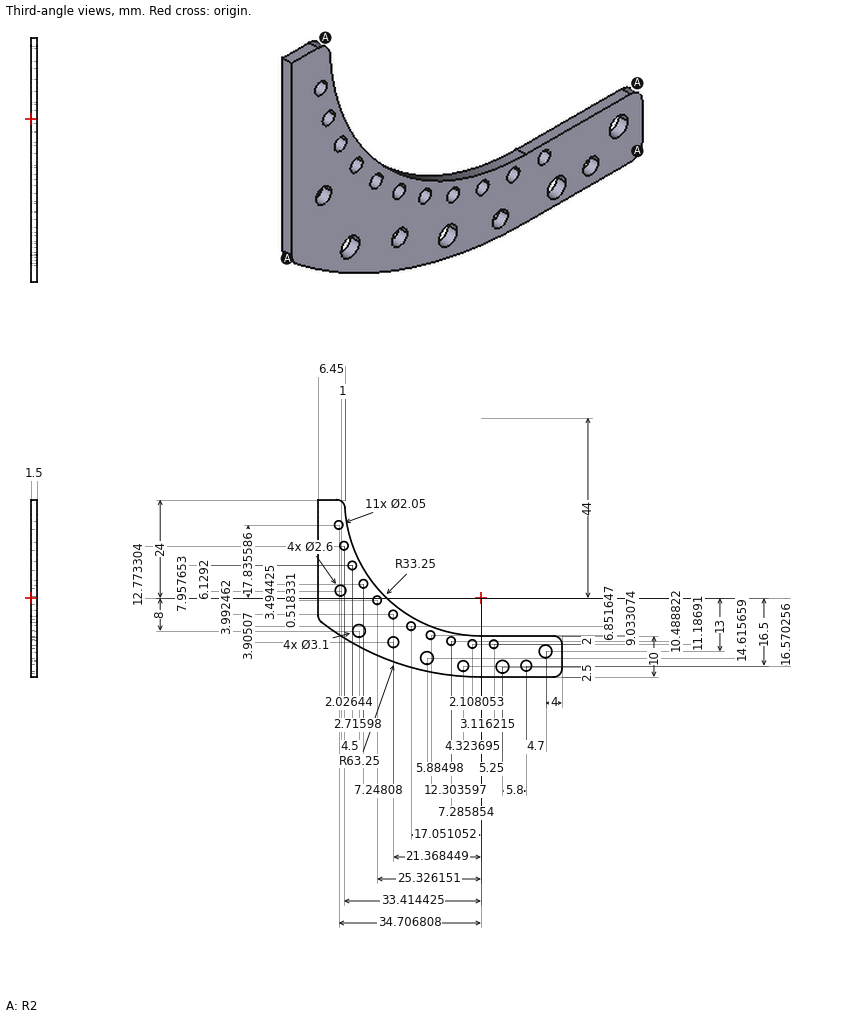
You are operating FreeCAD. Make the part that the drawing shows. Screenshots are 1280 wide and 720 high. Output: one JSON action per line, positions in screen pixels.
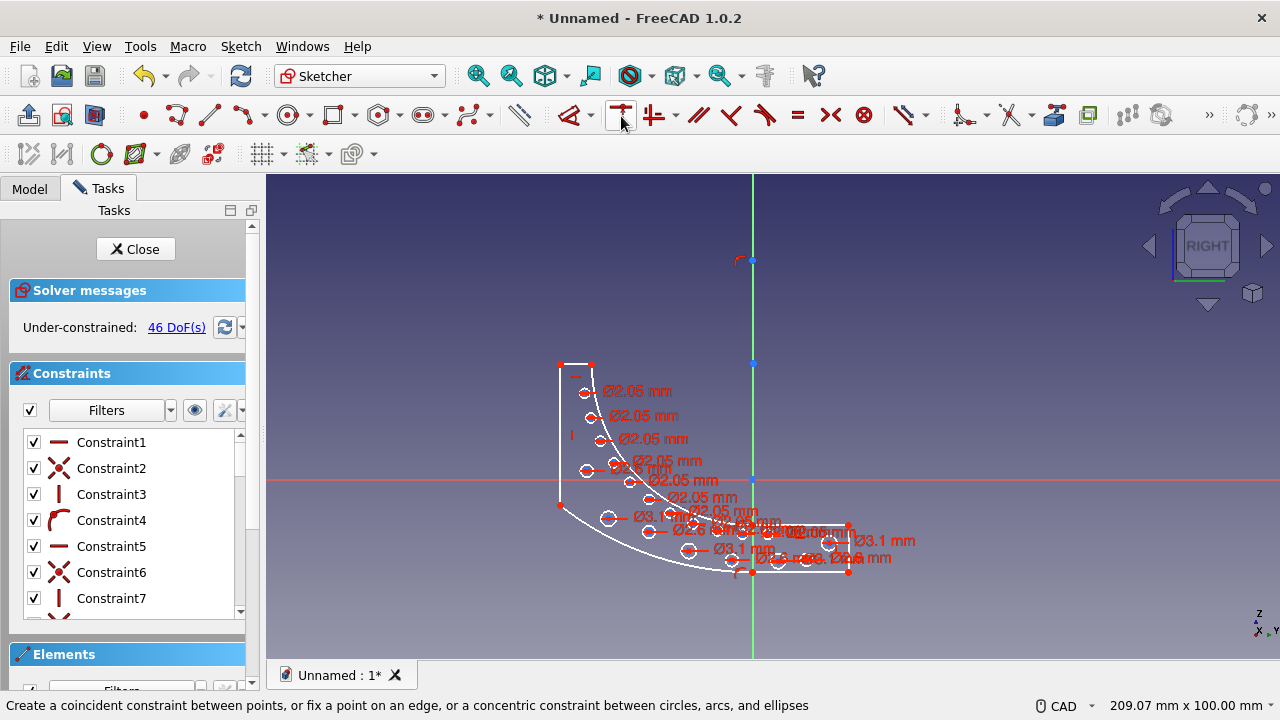
{"action": "left_click", "coordinate": [753, 364]}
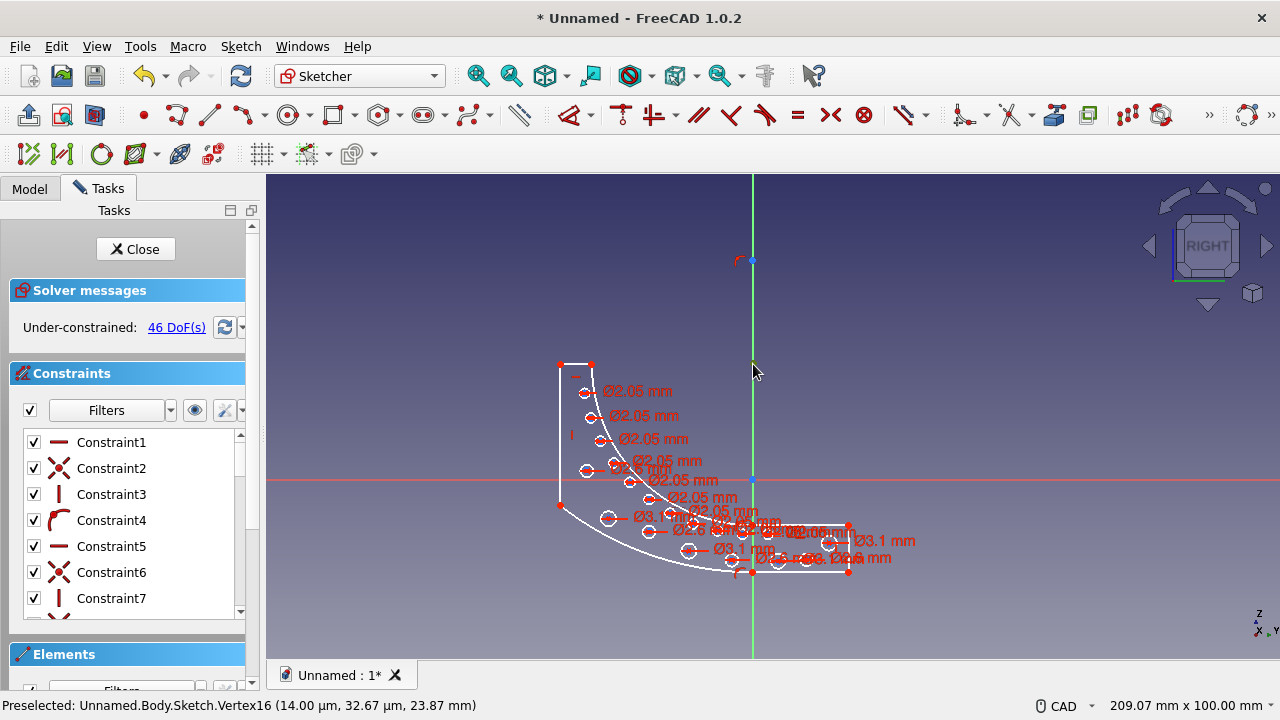
{"action": "left_click", "coordinate": [753, 447]}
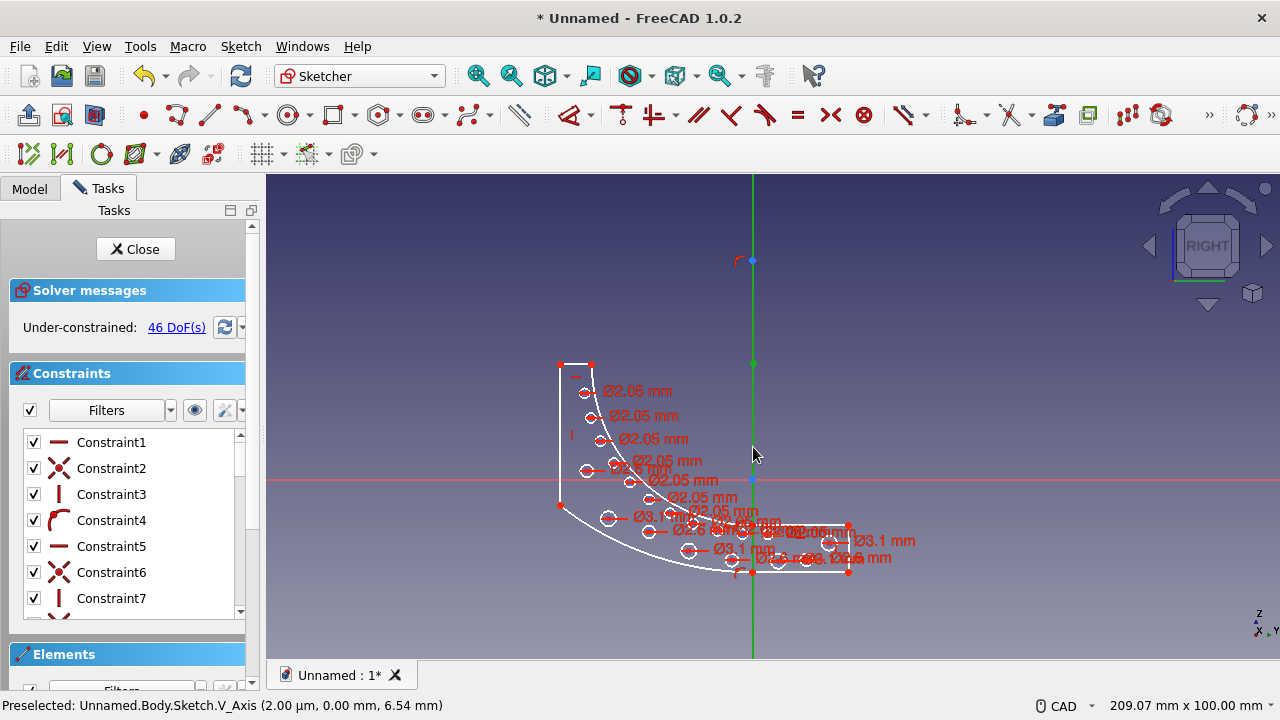
{"action": "left_click", "coordinate": [621, 116]}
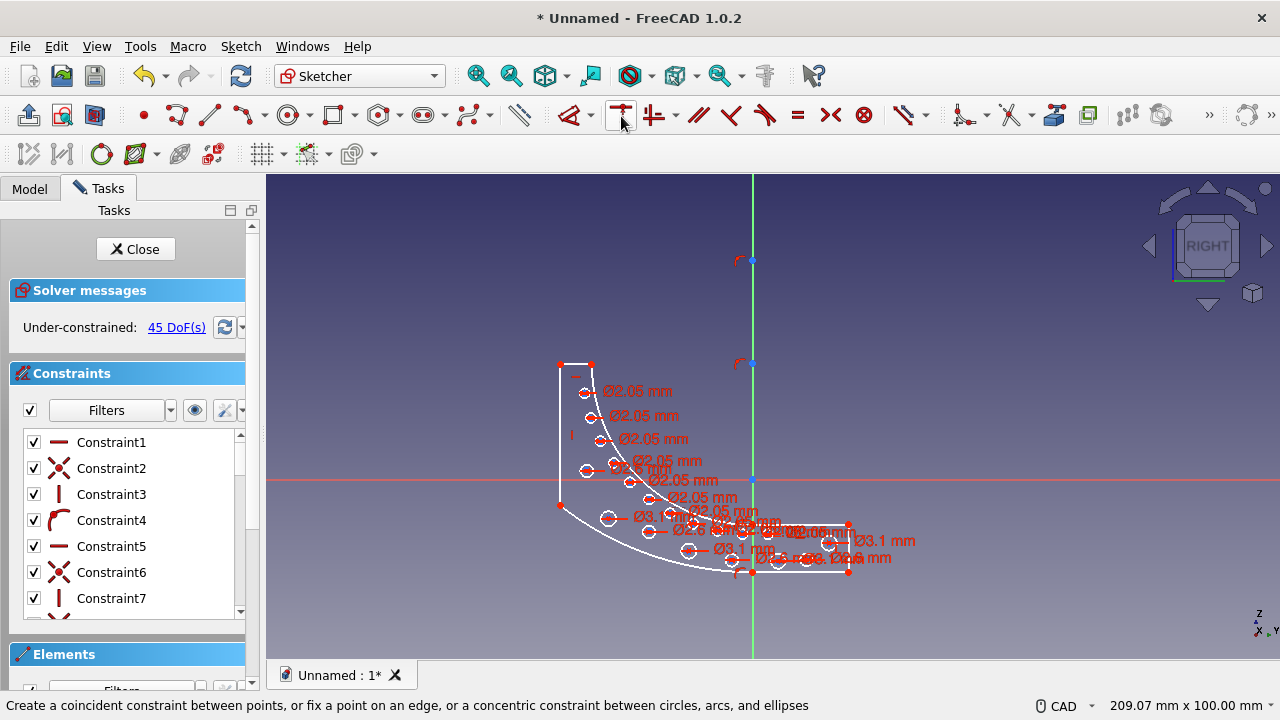
{"action": "left_click", "coordinate": [568, 116]}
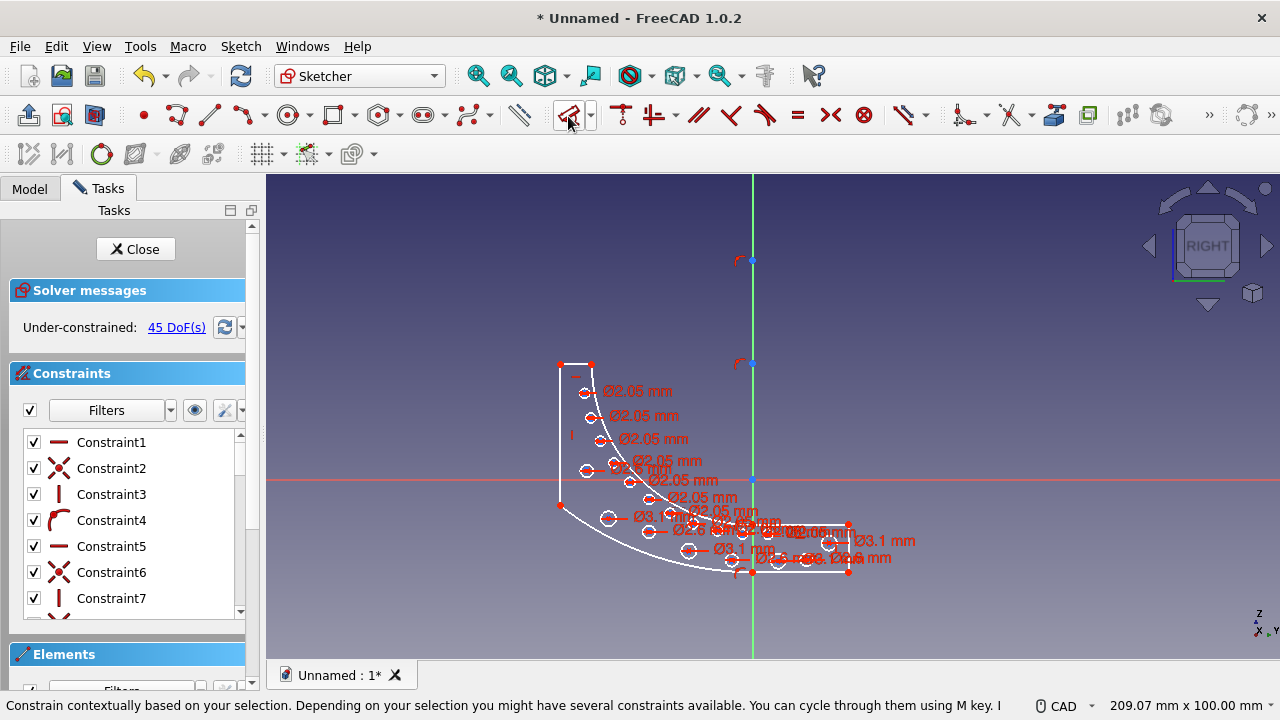
{"action": "left_click", "coordinate": [613, 539]}
{"action": "left_click", "coordinate": [599, 568]}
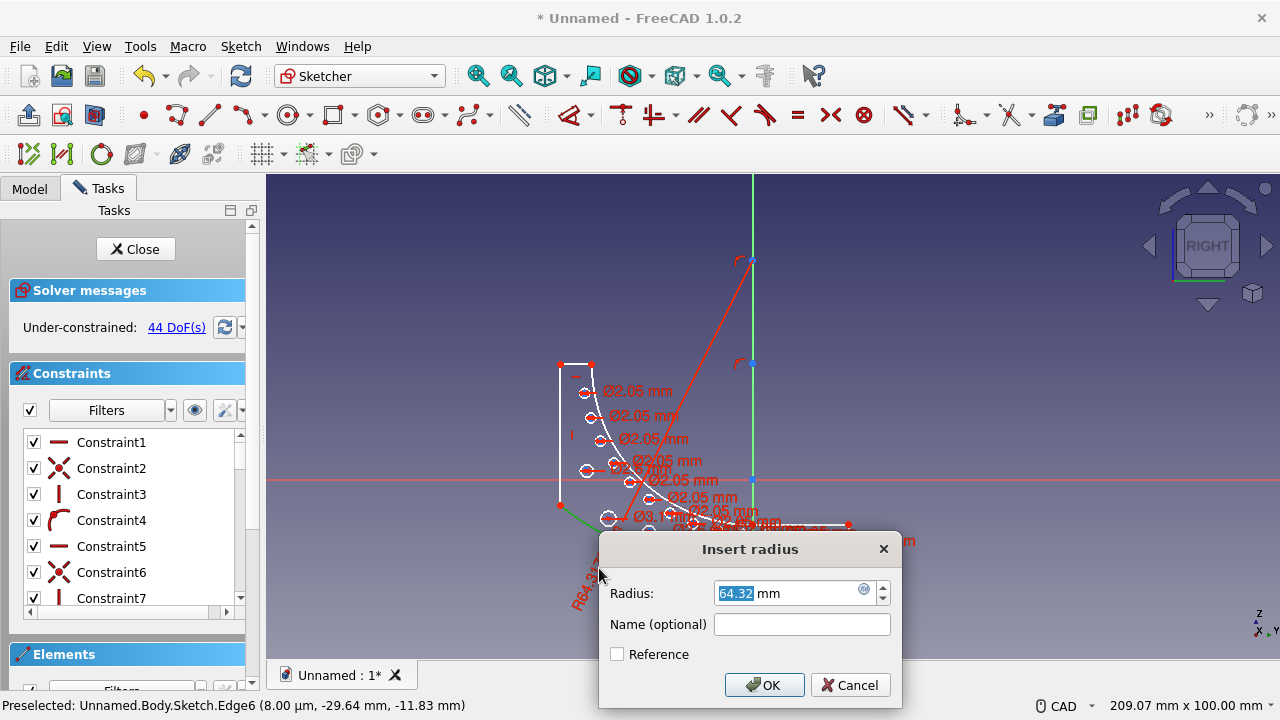
{"action": "type", "text": "63.25"}
{"action": "key", "text": "Return"}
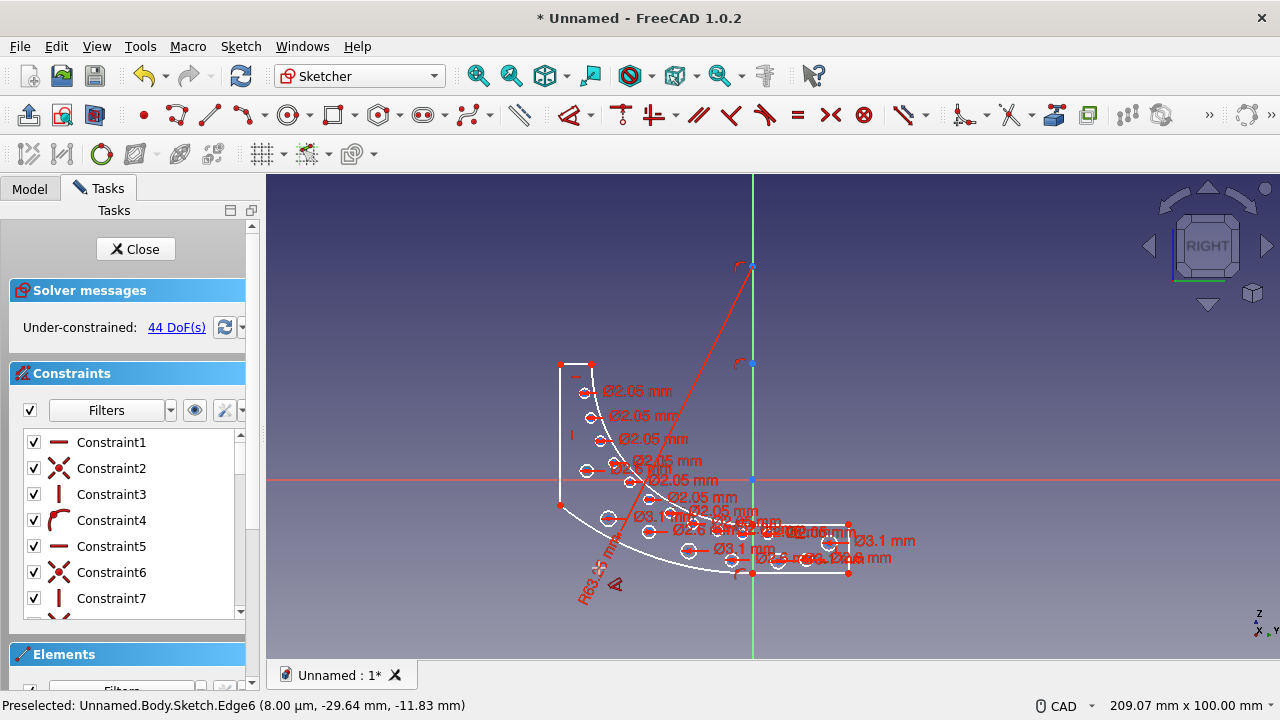
{"action": "scroll", "coordinate": [703, 517], "scroll_direction": "up", "scroll_amount": 4}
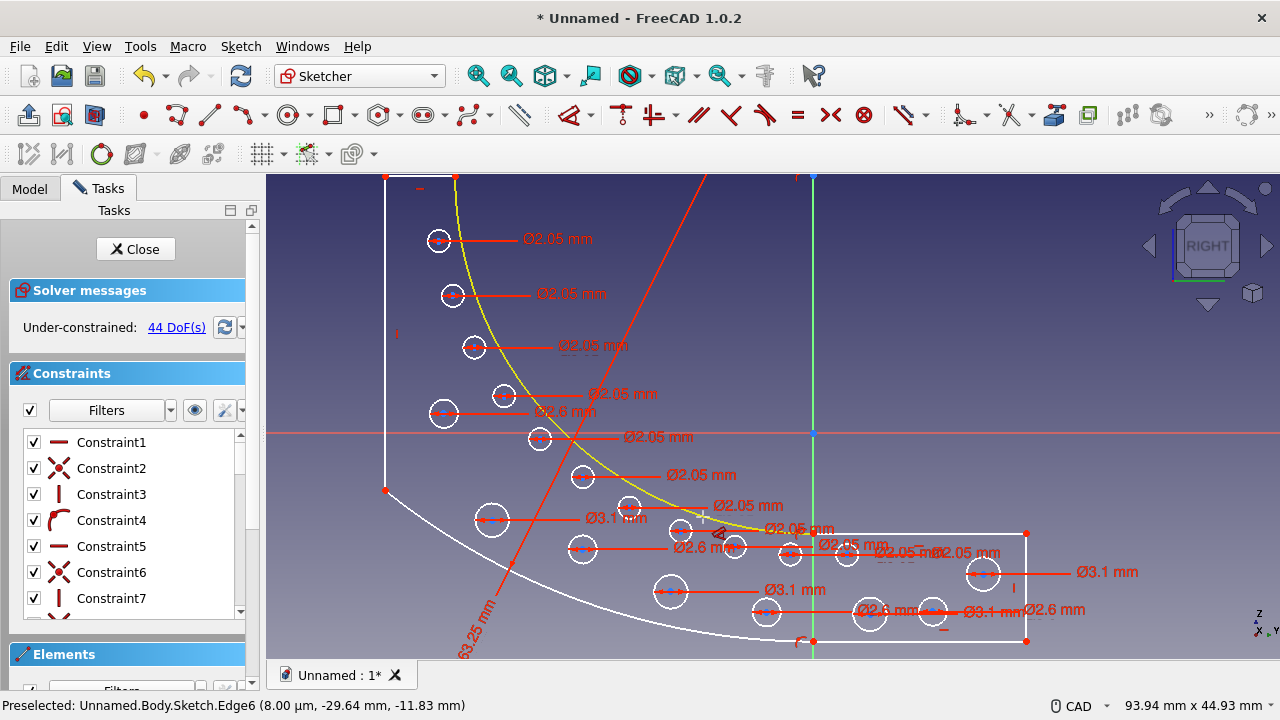
{"action": "left_click", "coordinate": [703, 516]}
{"action": "left_click", "coordinate": [886, 559]}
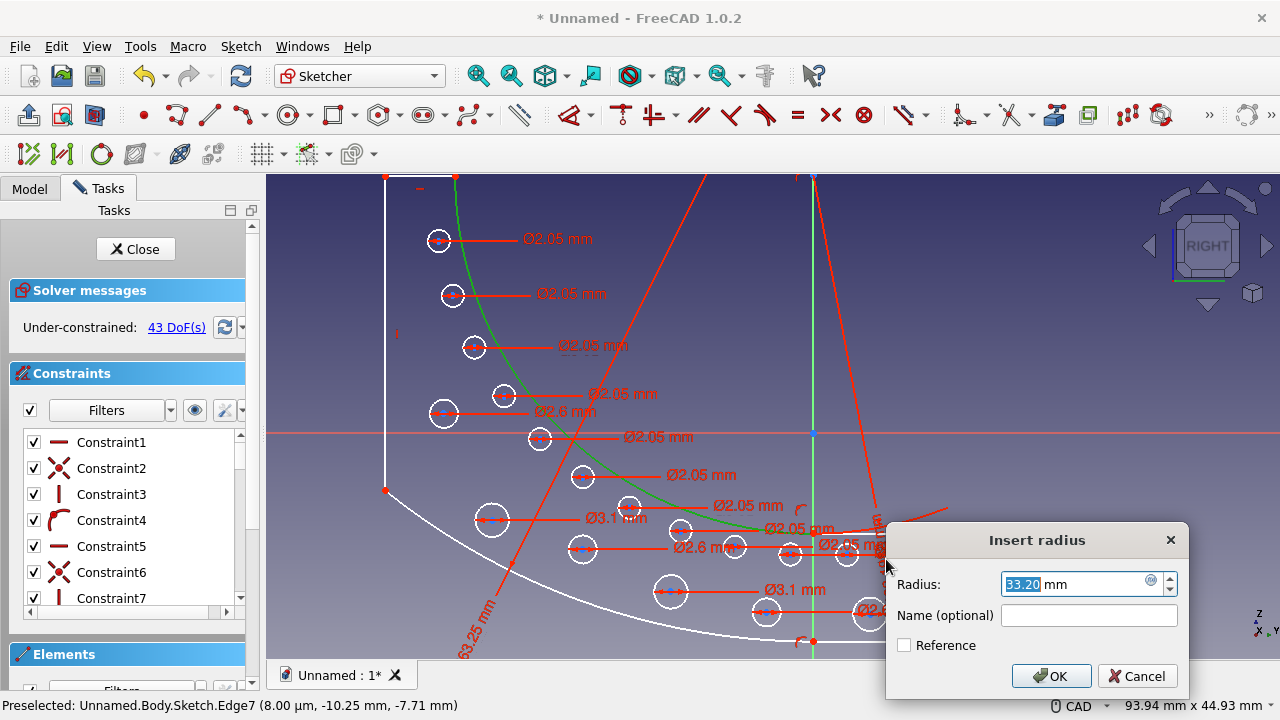
{"action": "type", "text": "33.25"}
{"action": "key", "text": "Return"}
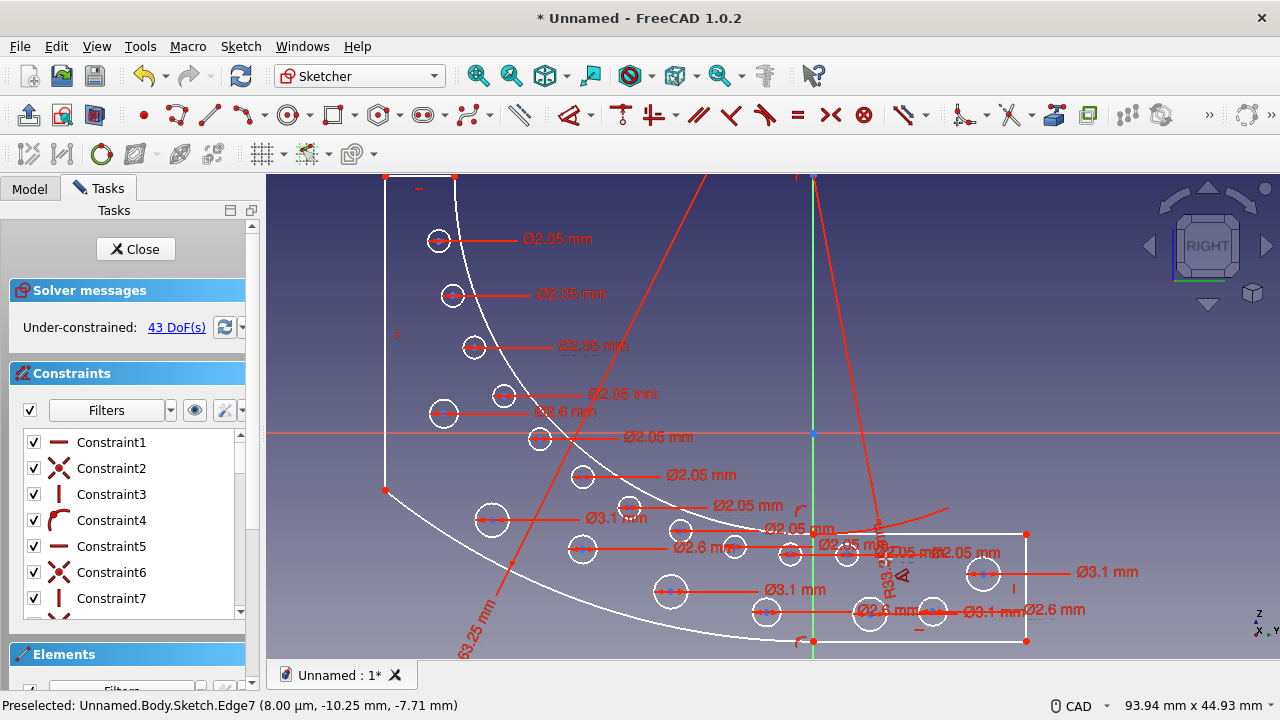
{"action": "left_click", "coordinate": [492, 520]}
{"action": "left_click", "coordinate": [458, 477]}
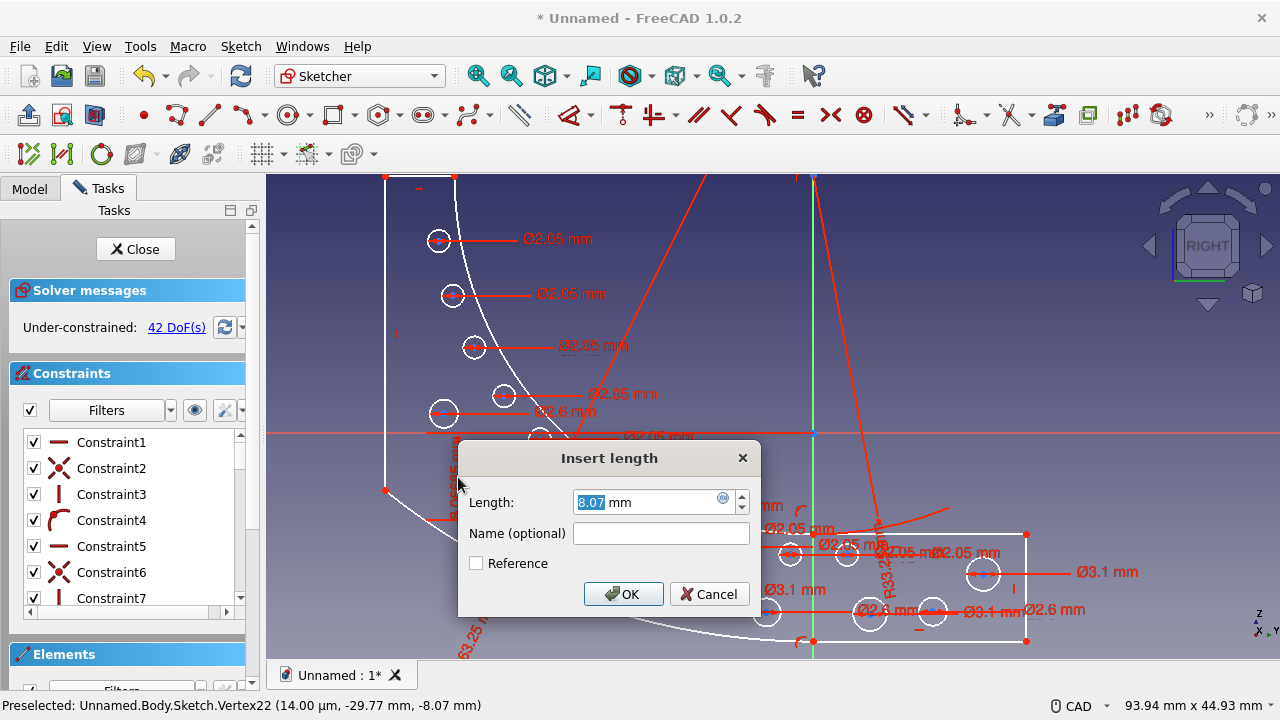
{"action": "type", "text": "8"}
{"action": "key", "text": "Return"}